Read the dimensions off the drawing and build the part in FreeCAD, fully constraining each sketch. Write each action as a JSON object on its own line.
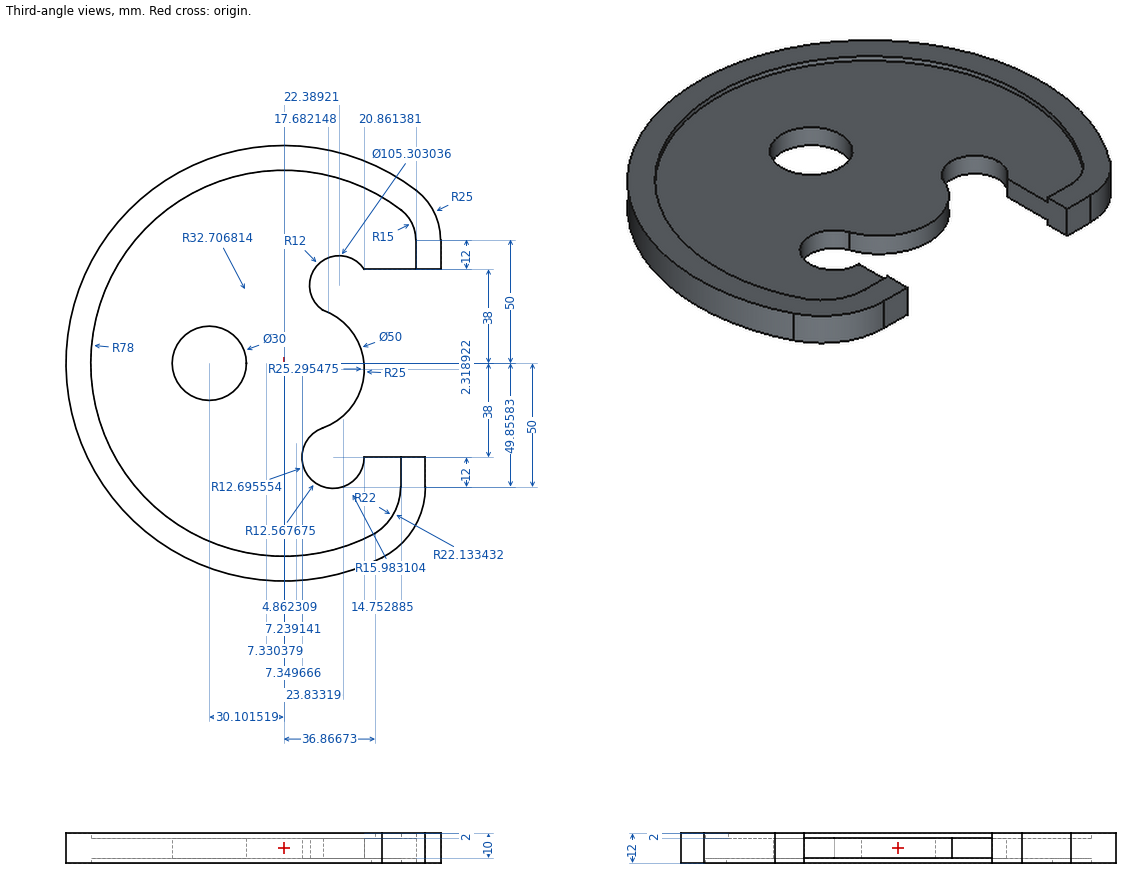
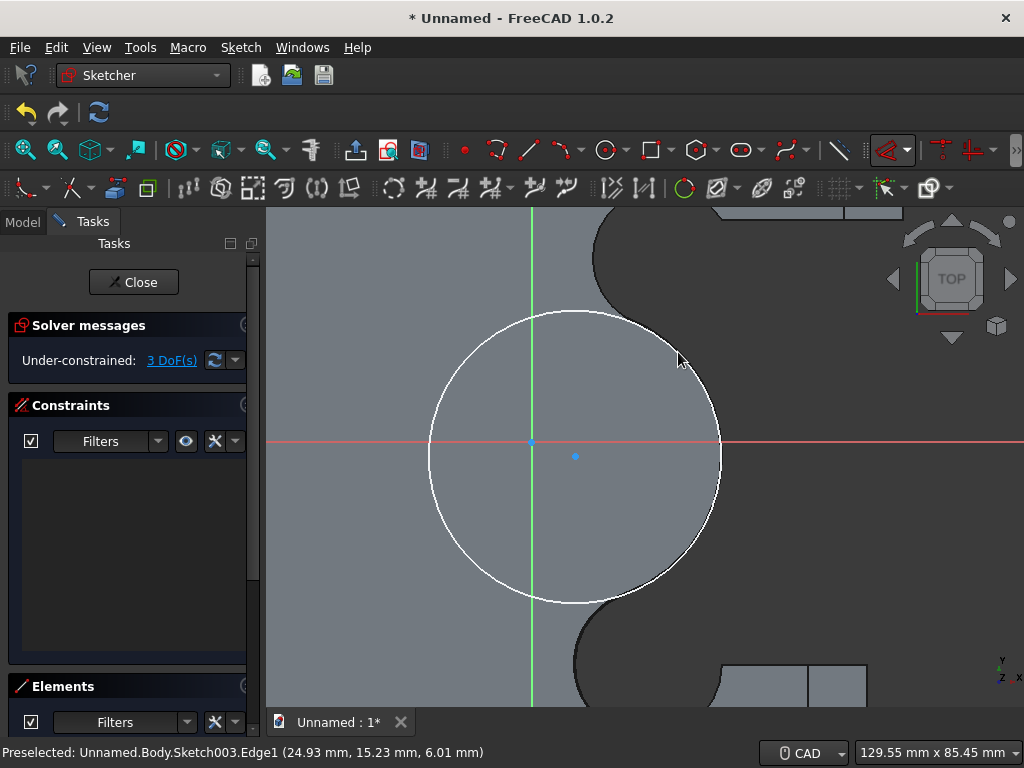
{"action": "left_click", "coordinate": [678, 353]}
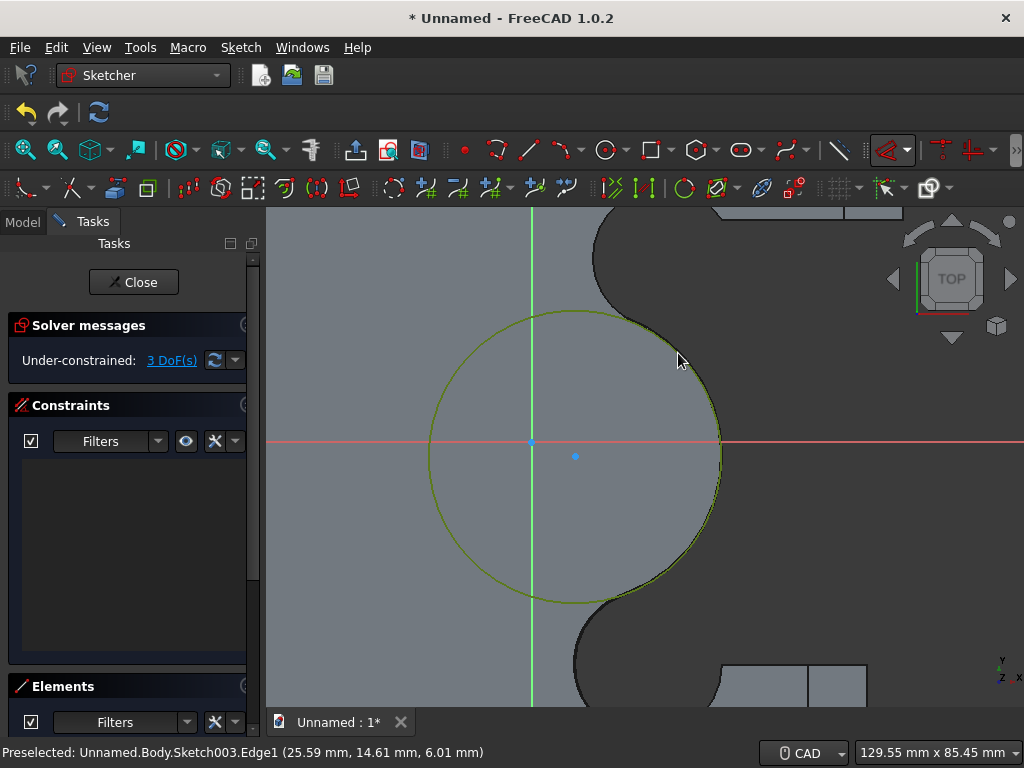
{"action": "key", "text": "k o"}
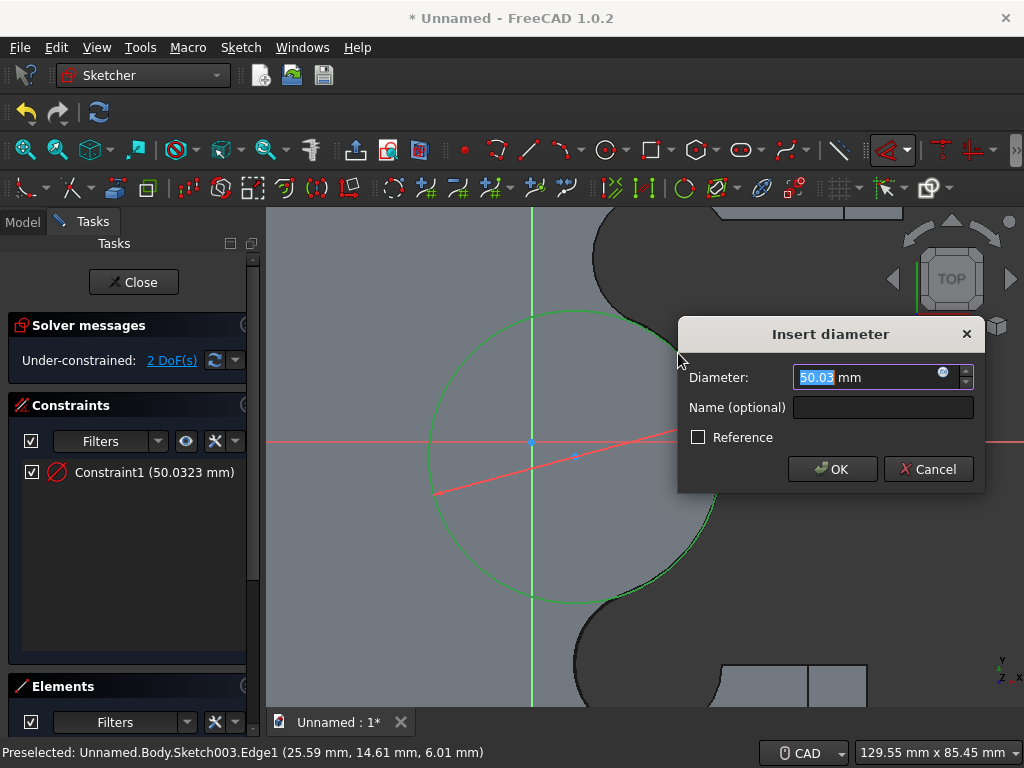
{"action": "type", "text": "50"}
{"action": "key", "text": "Return"}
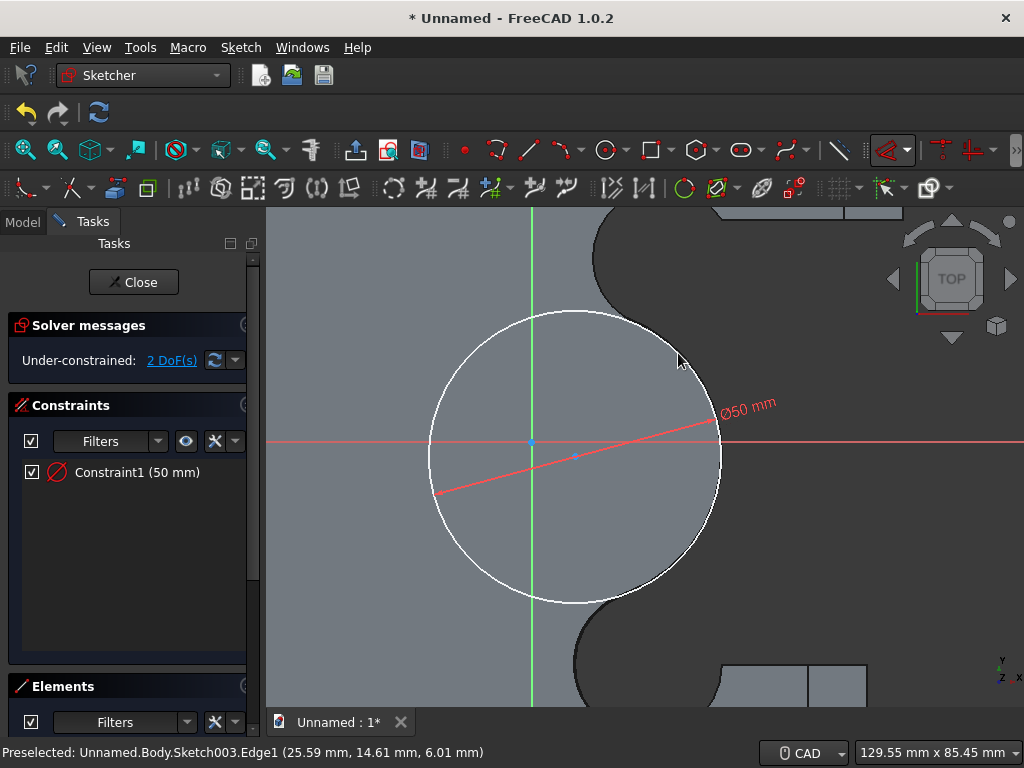
{"action": "left_click", "coordinate": [575, 457]}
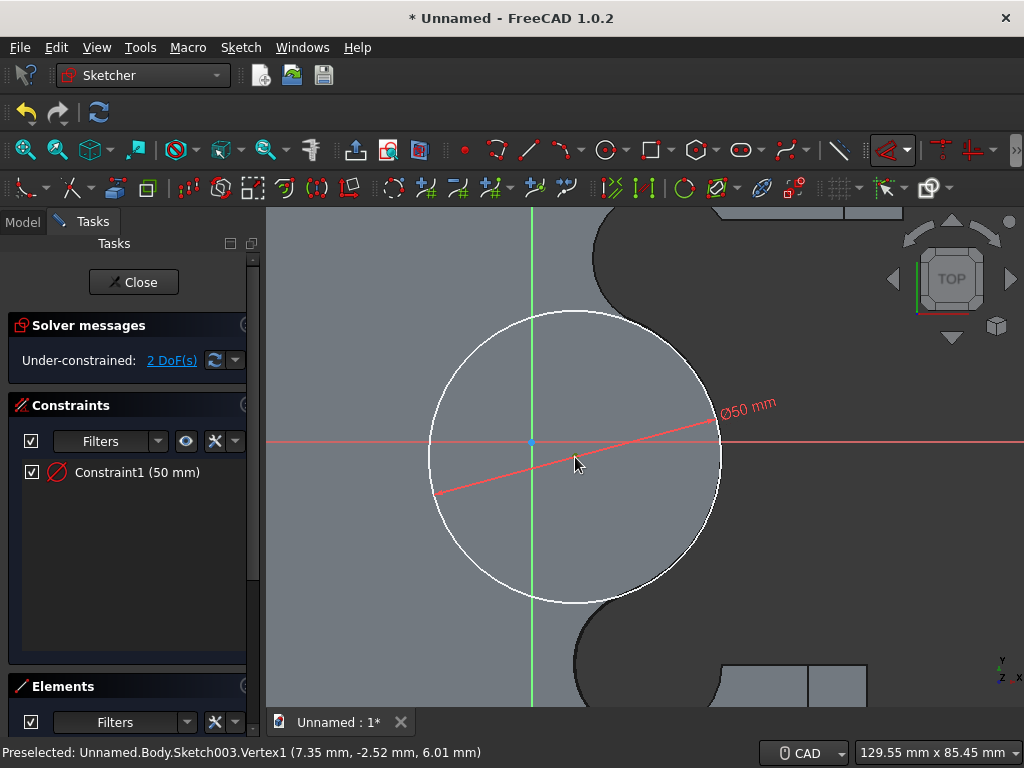
{"action": "left_click", "coordinate": [910, 150]}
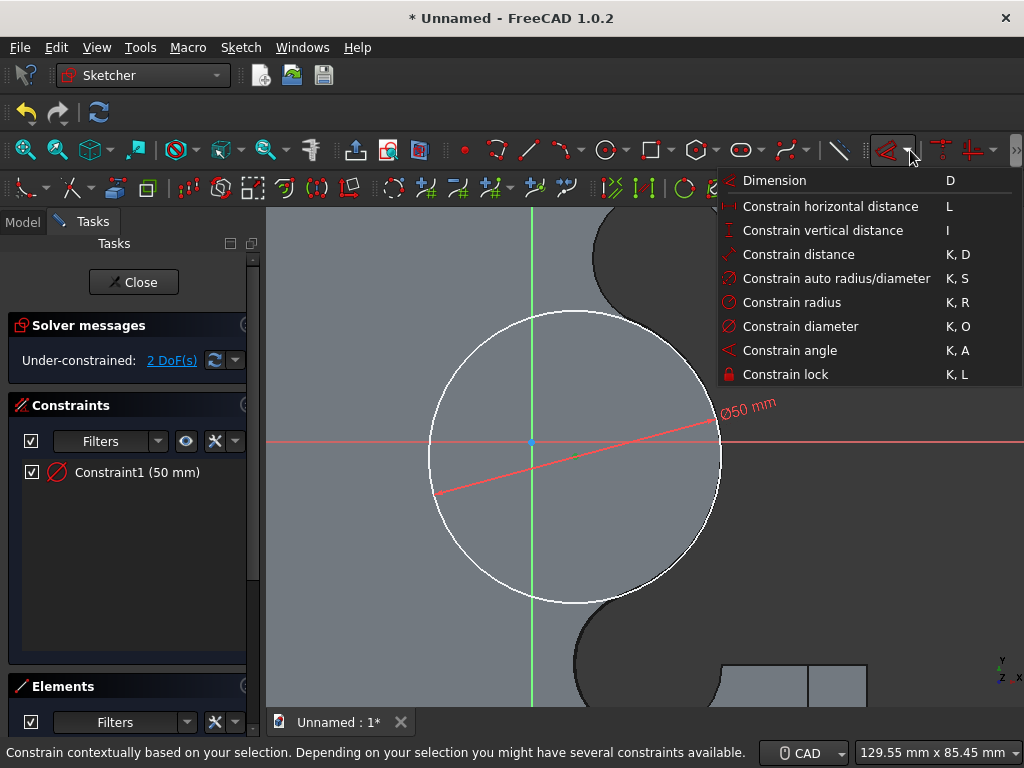
{"action": "left_click", "coordinate": [870, 206]}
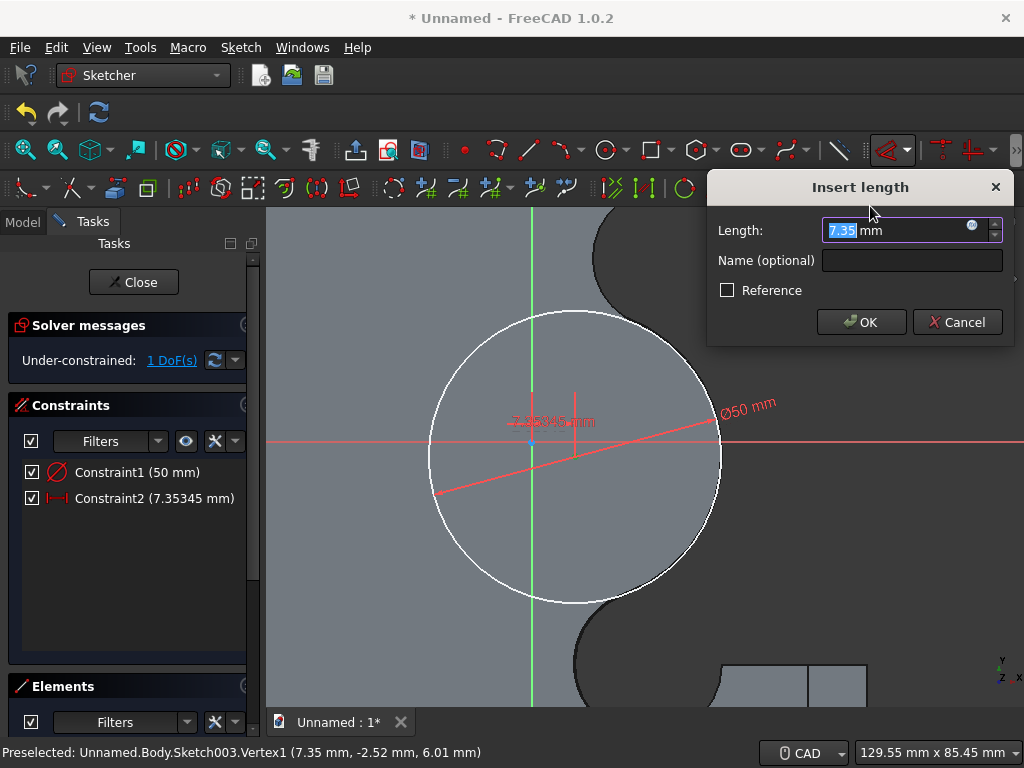
{"action": "type", "text": "7.349666"}
{"action": "key", "text": "Return"}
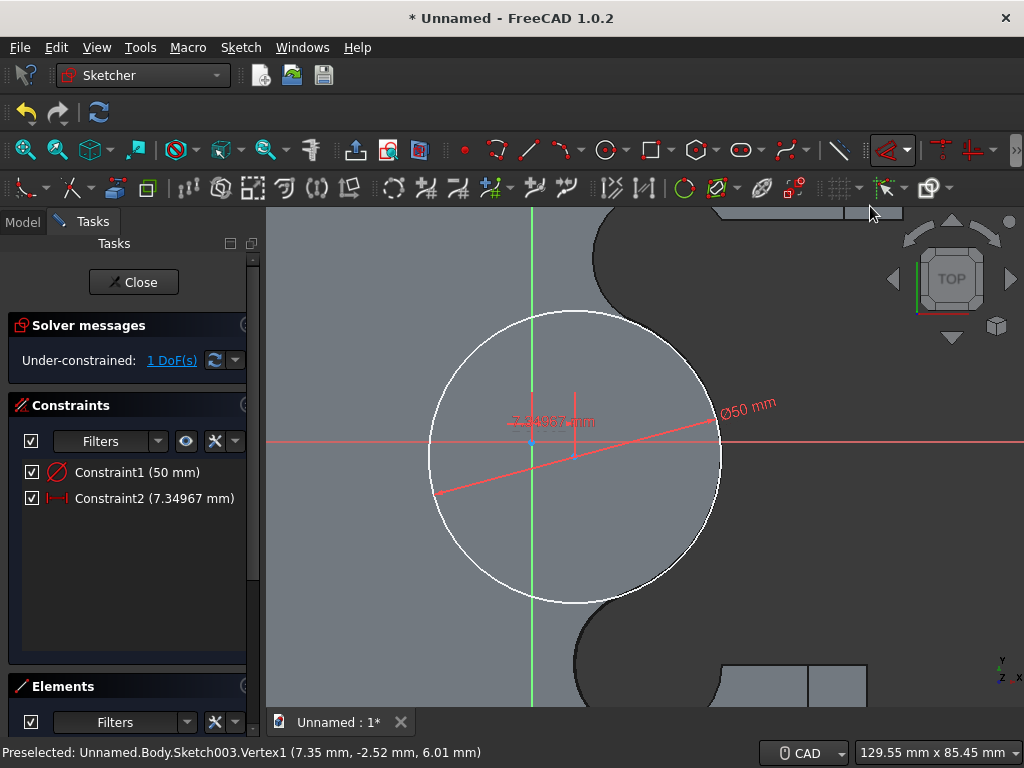
{"action": "scroll", "coordinate": [575, 457], "scroll_direction": "up", "scroll_amount": 6}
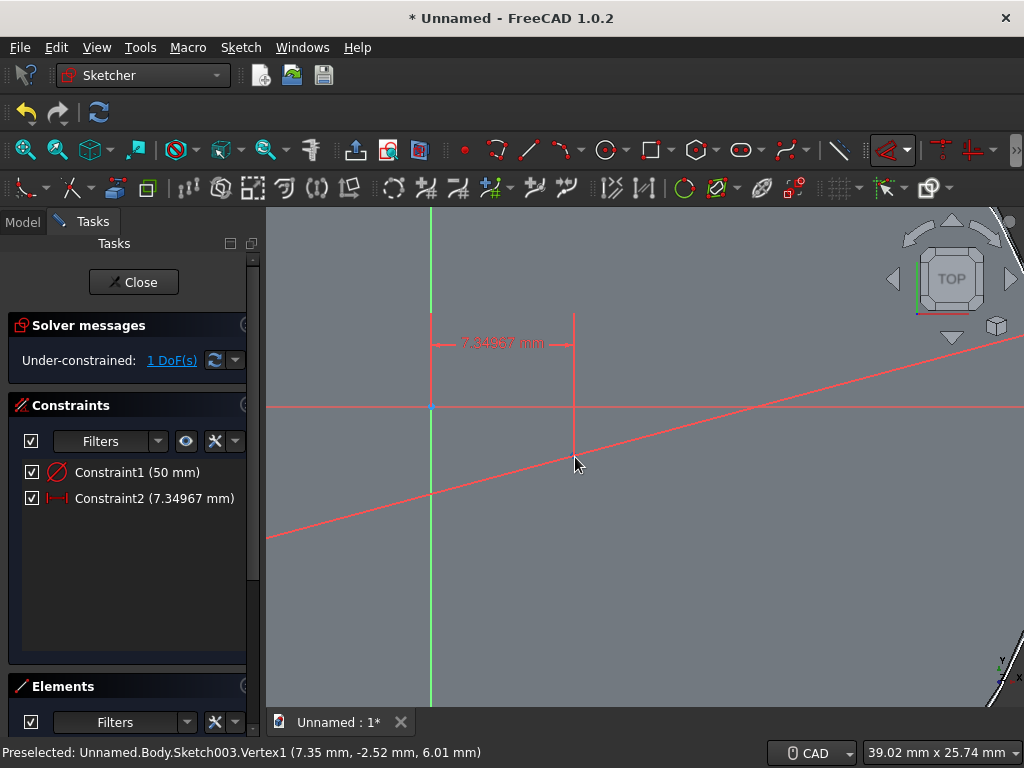
{"action": "left_click", "coordinate": [574, 456]}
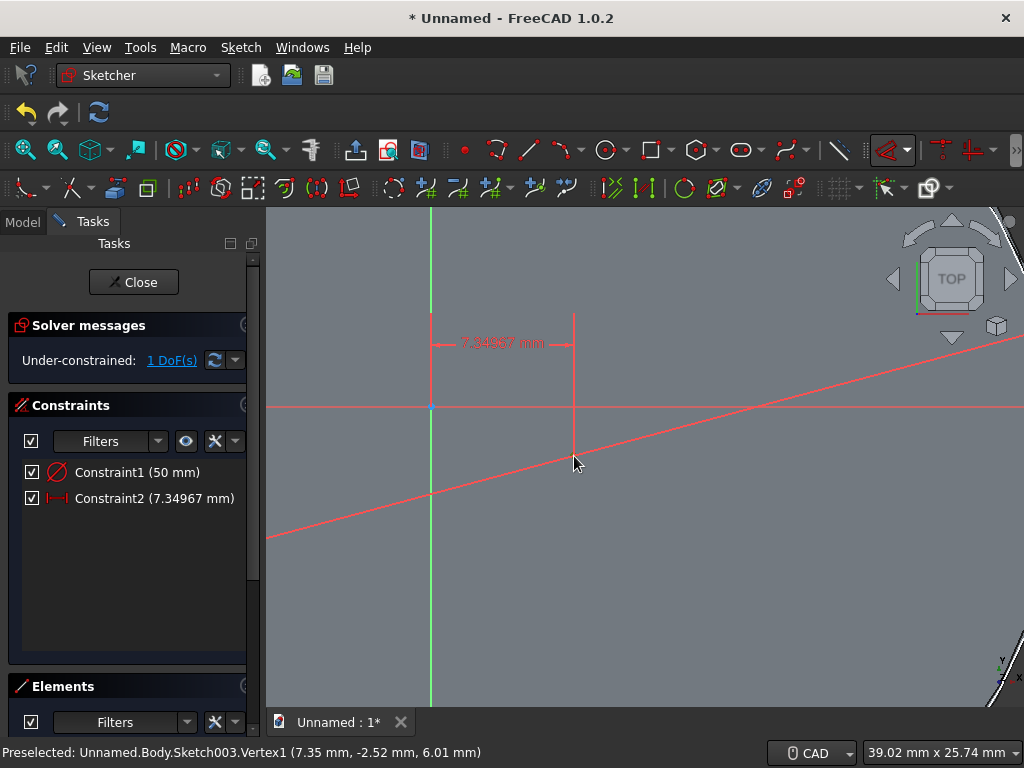
{"action": "key", "text": "i"}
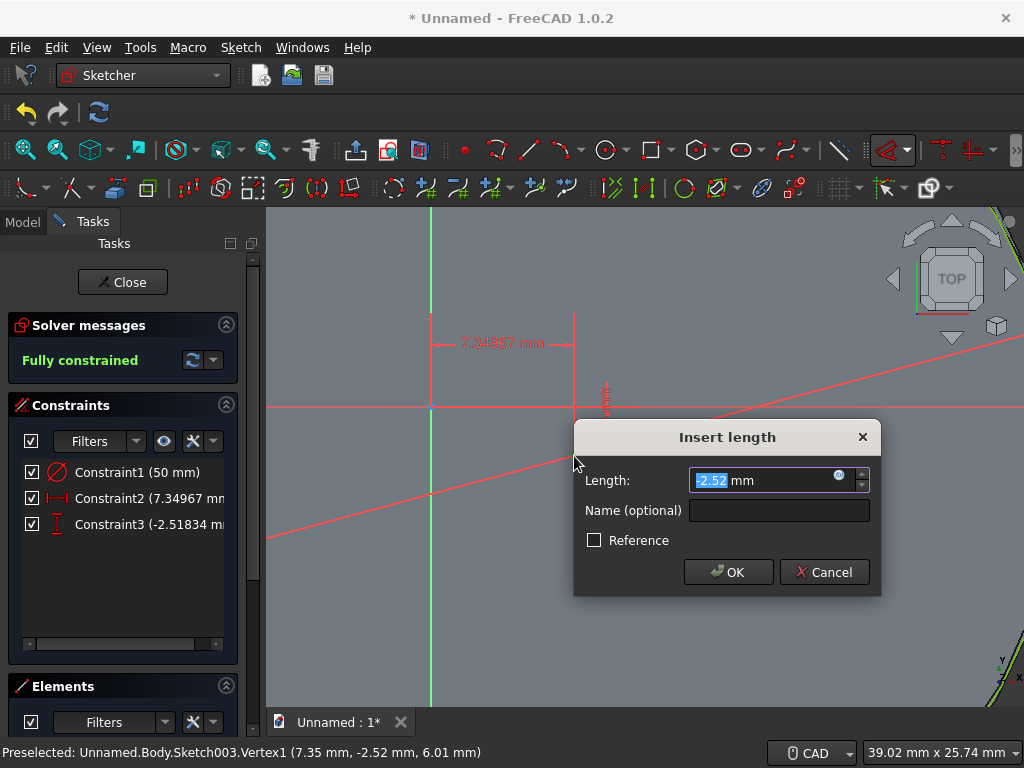
{"action": "type", "text": "-2.318922"}
{"action": "key", "text": "Return"}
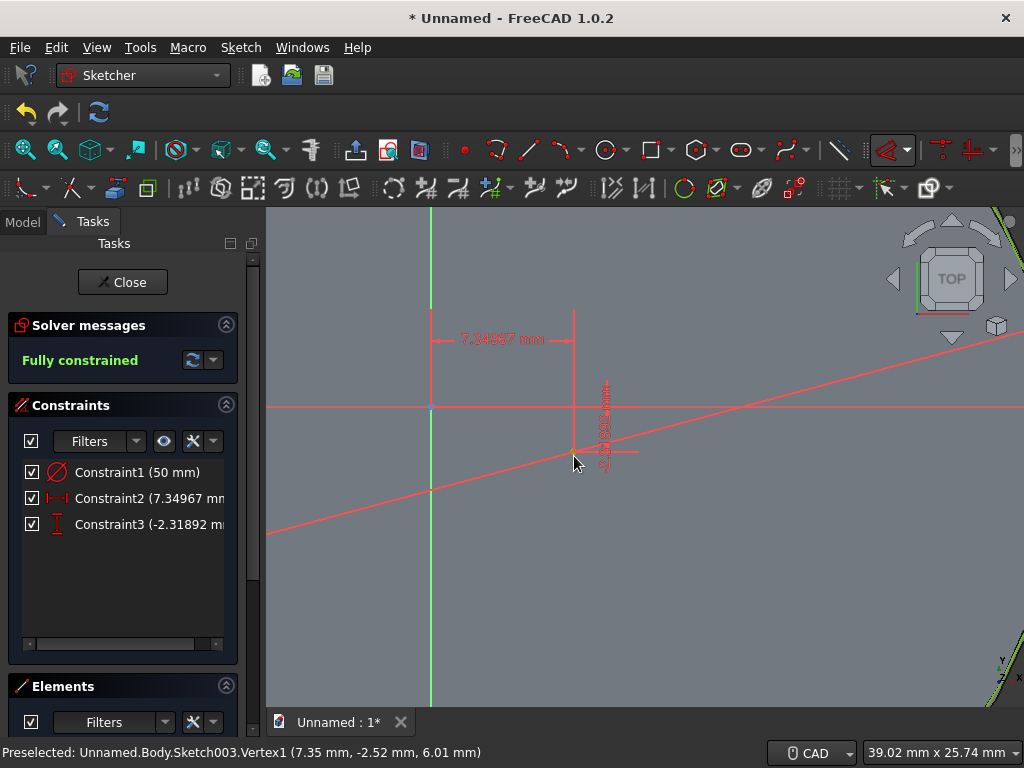
{"action": "left_click", "coordinate": [123, 282]}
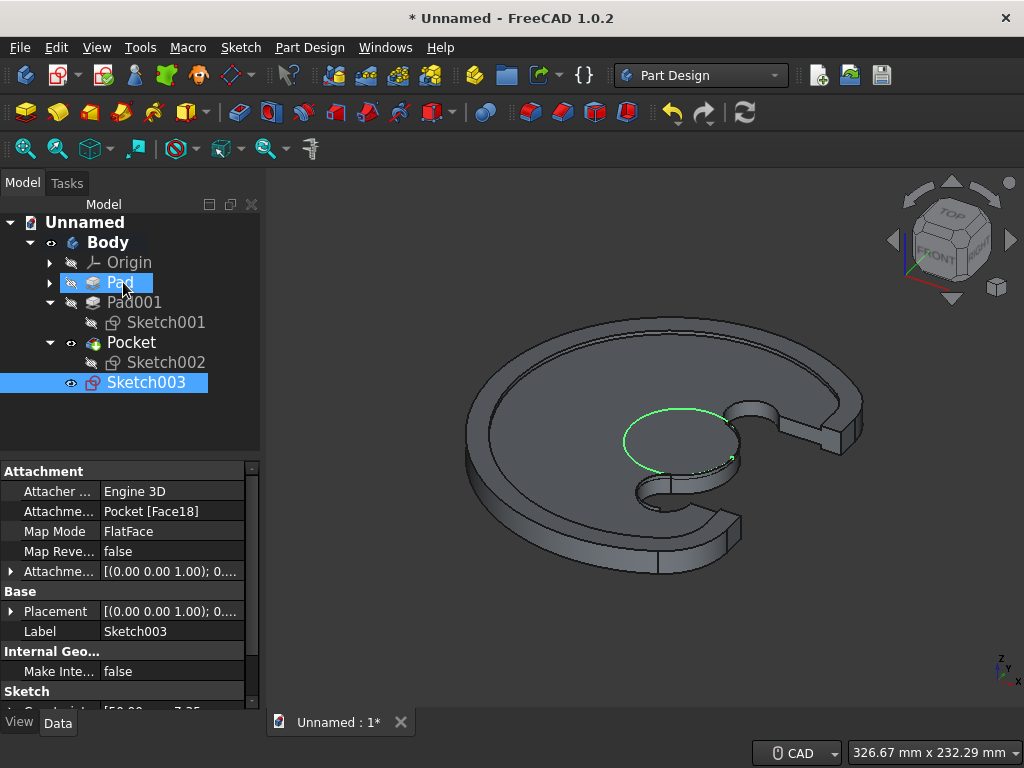
{"action": "left_click", "coordinate": [240, 112]}